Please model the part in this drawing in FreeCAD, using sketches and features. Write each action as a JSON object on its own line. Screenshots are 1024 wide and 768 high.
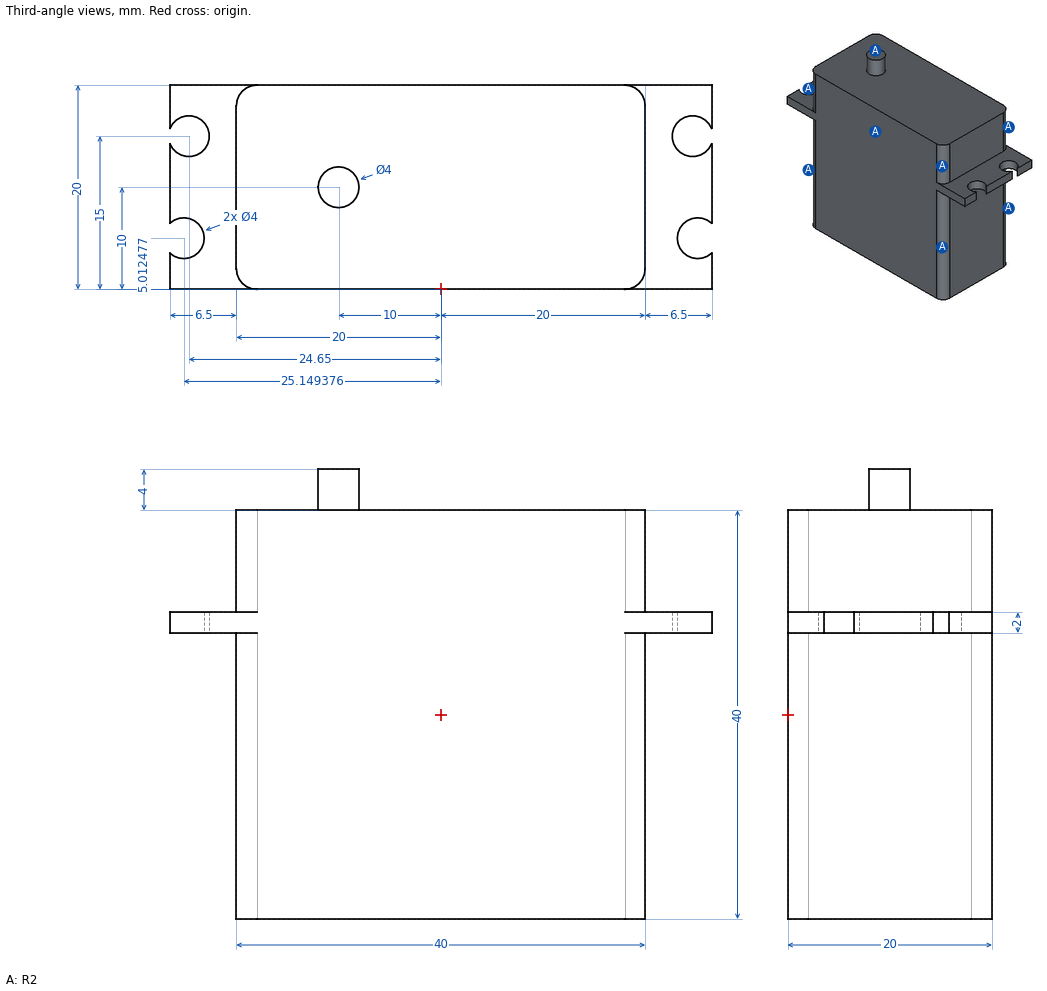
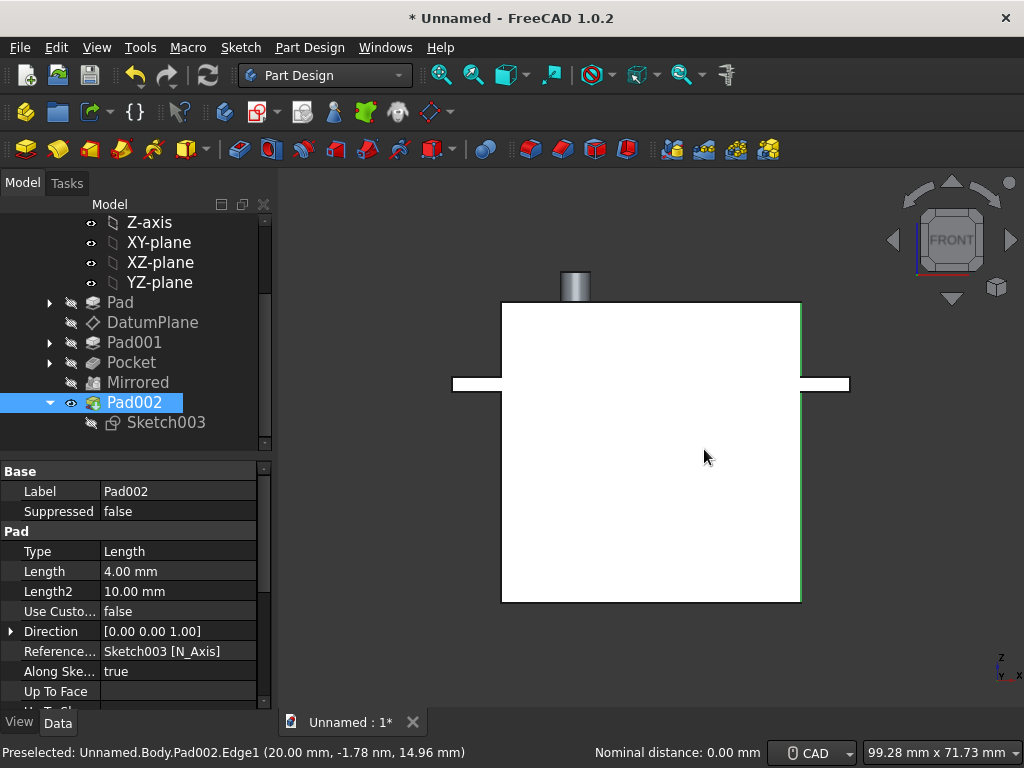
{"action": "left_click", "coordinate": [501, 339], "text": "ctrl"}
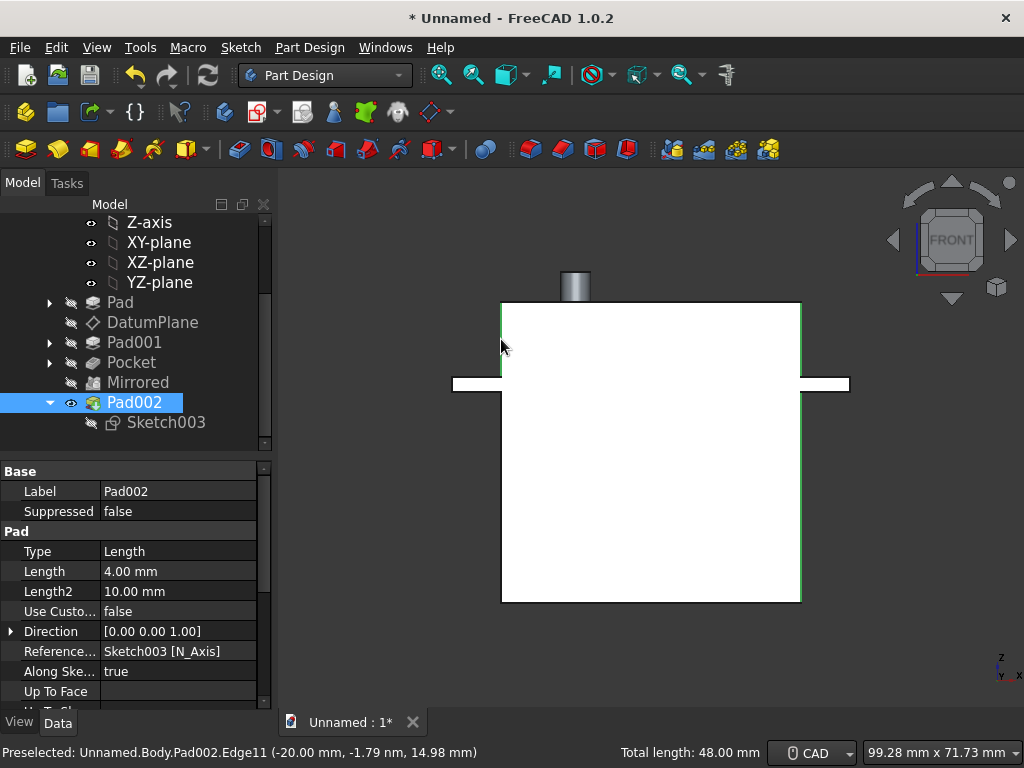
{"action": "left_click", "coordinate": [501, 497], "text": "ctrl"}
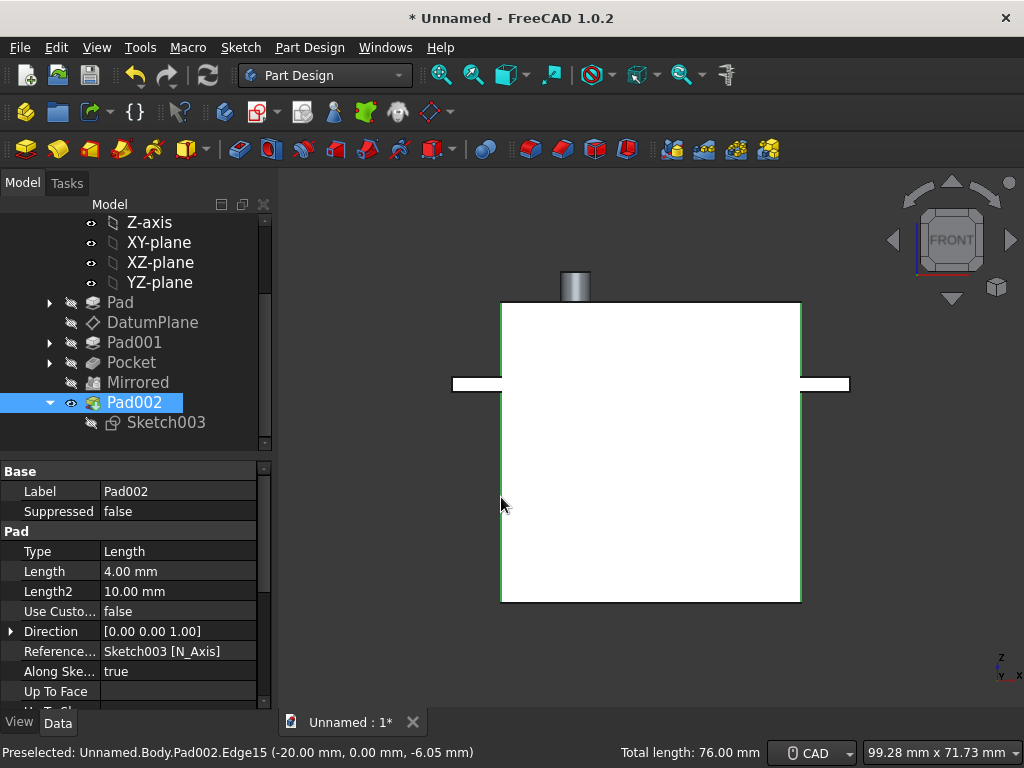
{"action": "key", "text": "3"}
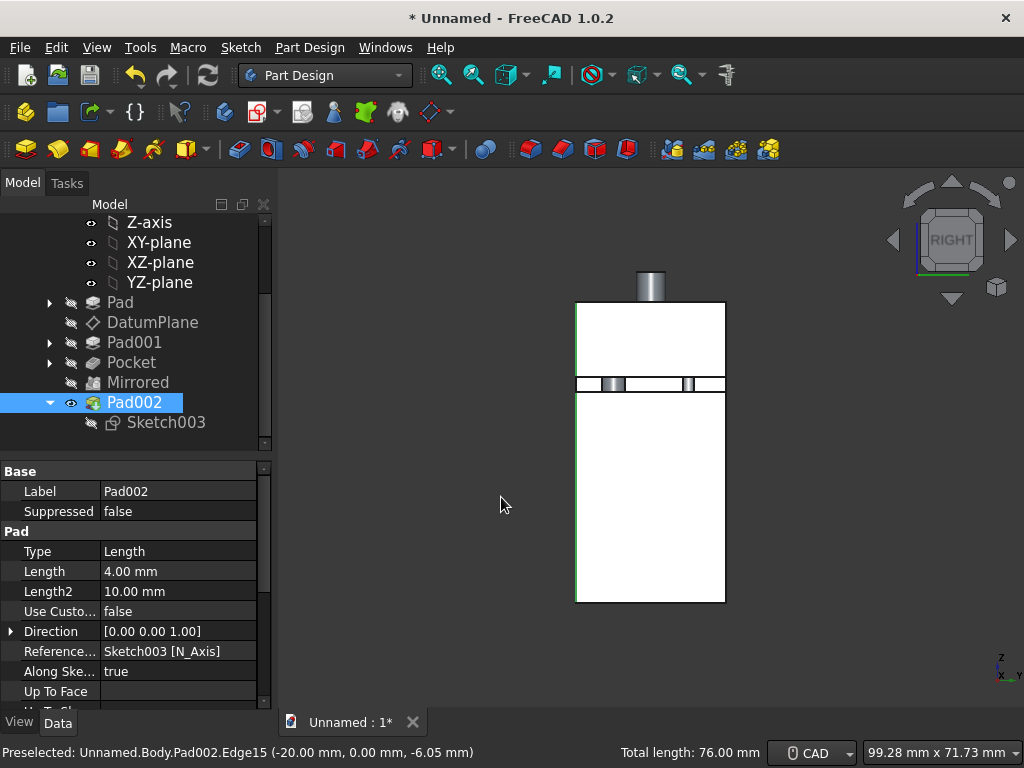
{"action": "left_click", "coordinate": [726, 497], "text": "ctrl"}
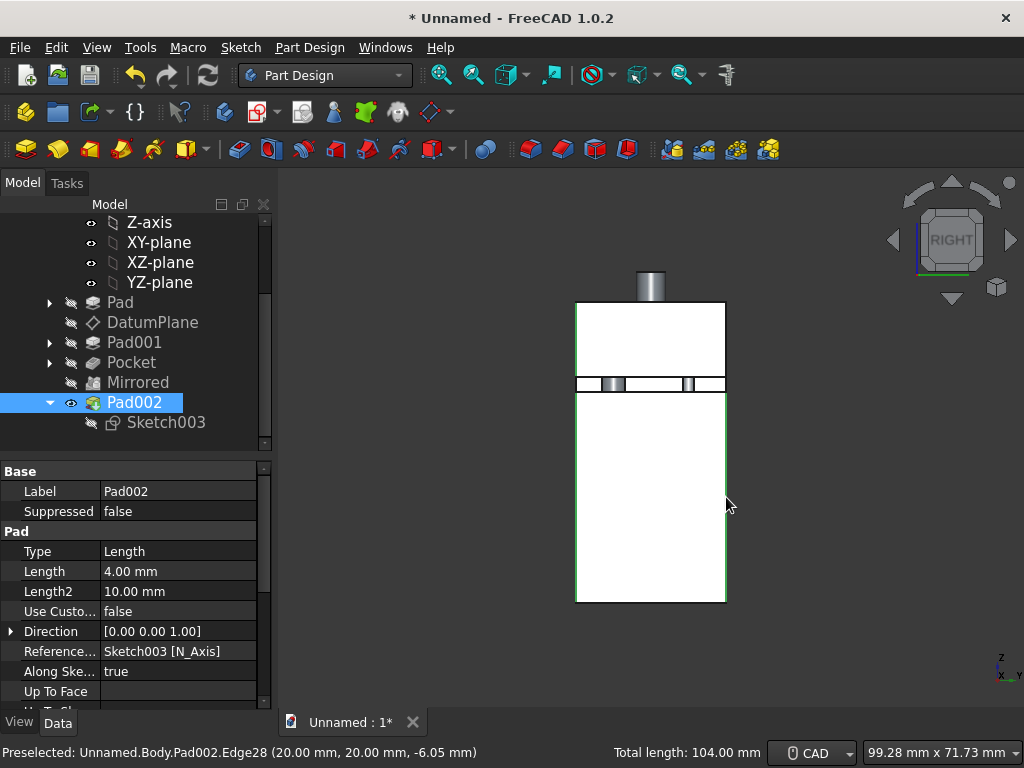
{"action": "left_click", "coordinate": [726, 339], "text": "ctrl"}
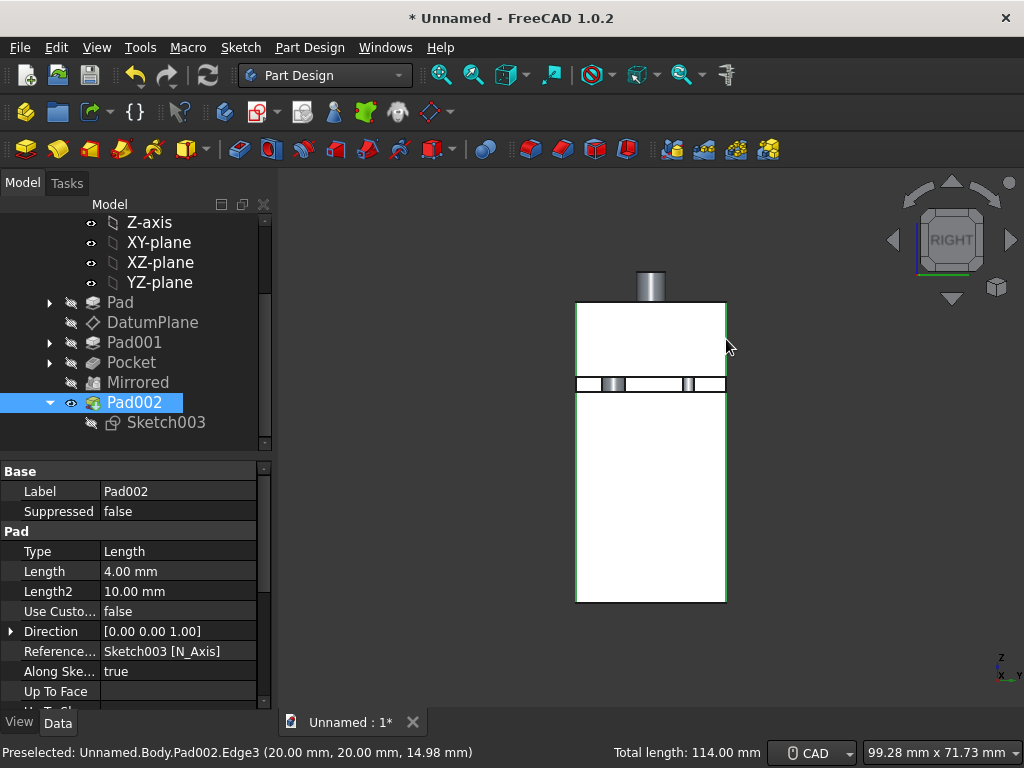
{"action": "key", "text": "5"}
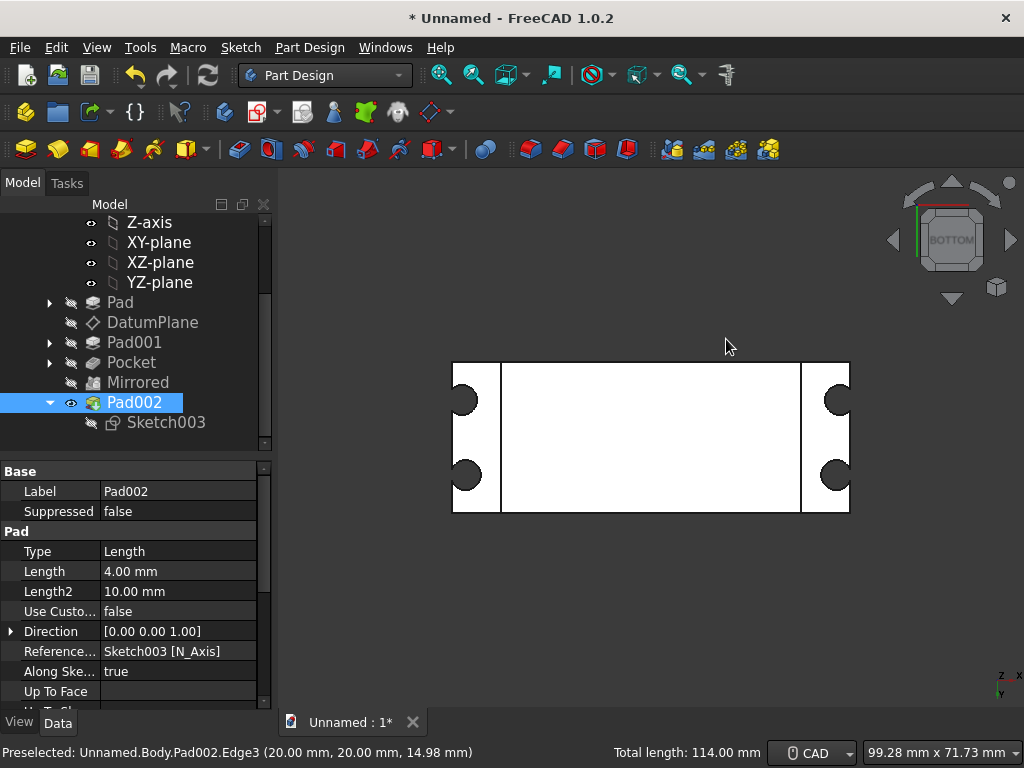
{"action": "key", "text": "4"}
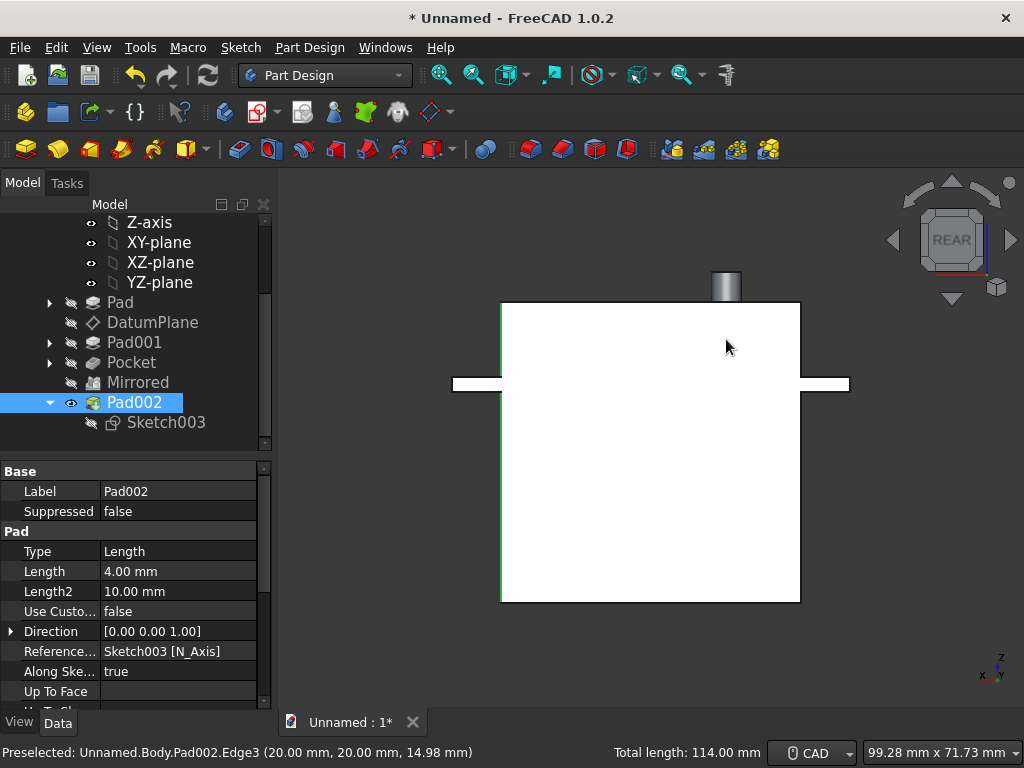
{"action": "left_click", "coordinate": [801, 339], "text": "ctrl"}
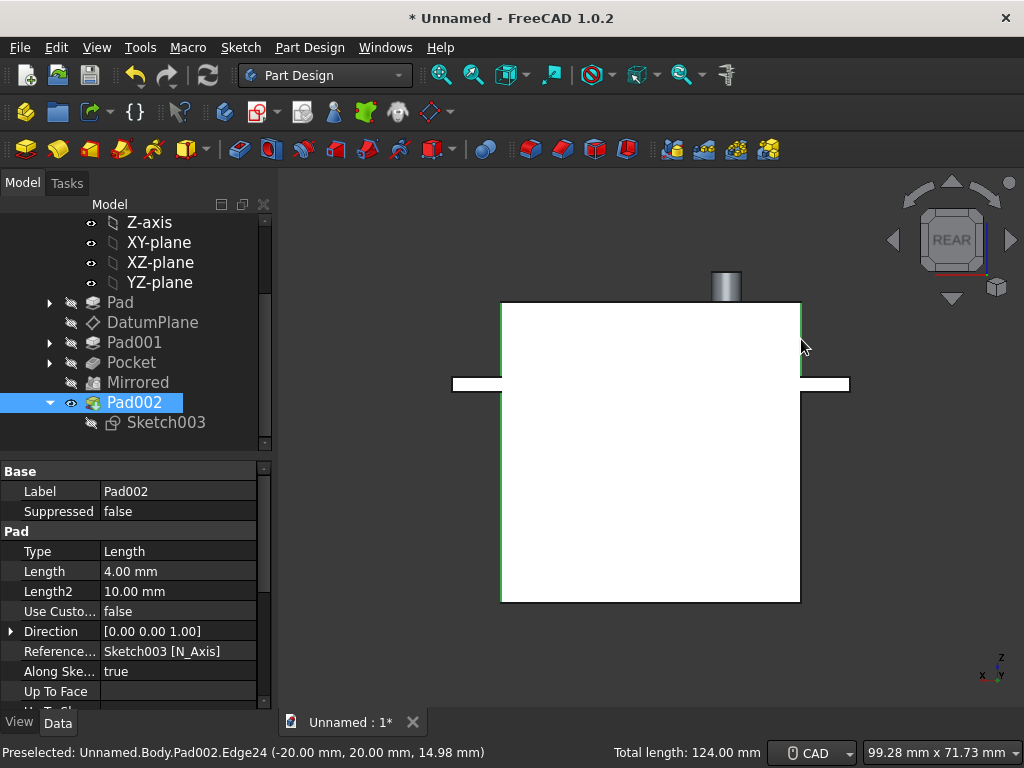
{"action": "left_click", "coordinate": [801, 497], "text": "ctrl"}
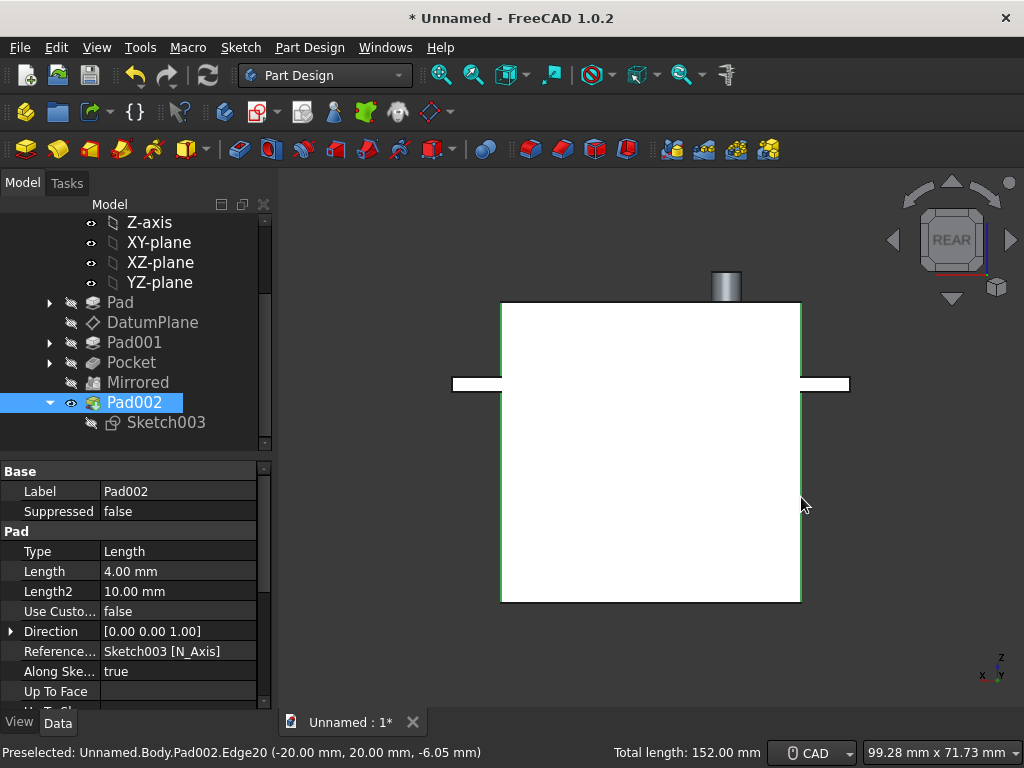
{"action": "left_click", "coordinate": [532, 150]}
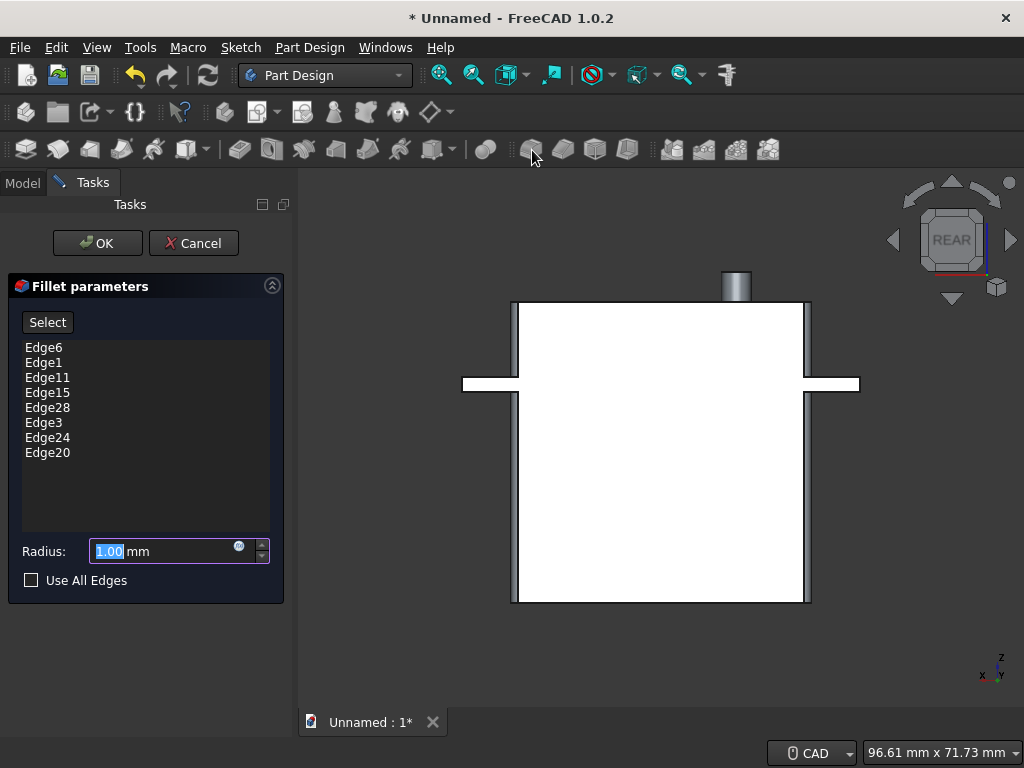
{"action": "type", "text": "2"}
{"action": "key", "text": "Tab"}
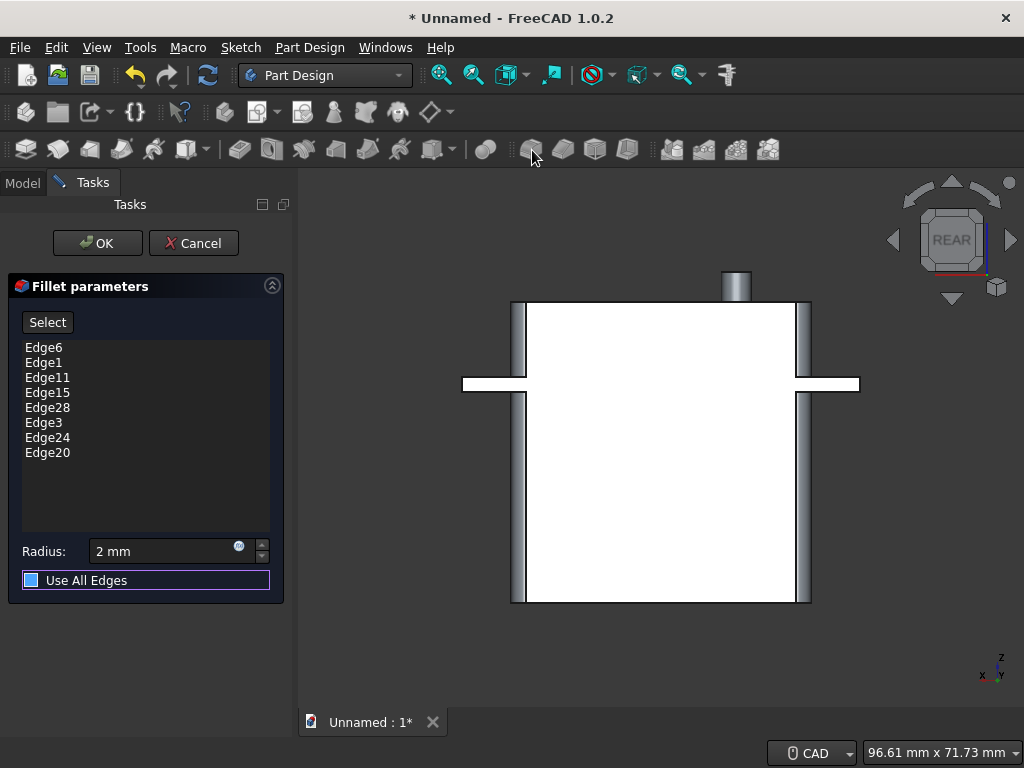
{"action": "left_click", "coordinate": [98, 243]}